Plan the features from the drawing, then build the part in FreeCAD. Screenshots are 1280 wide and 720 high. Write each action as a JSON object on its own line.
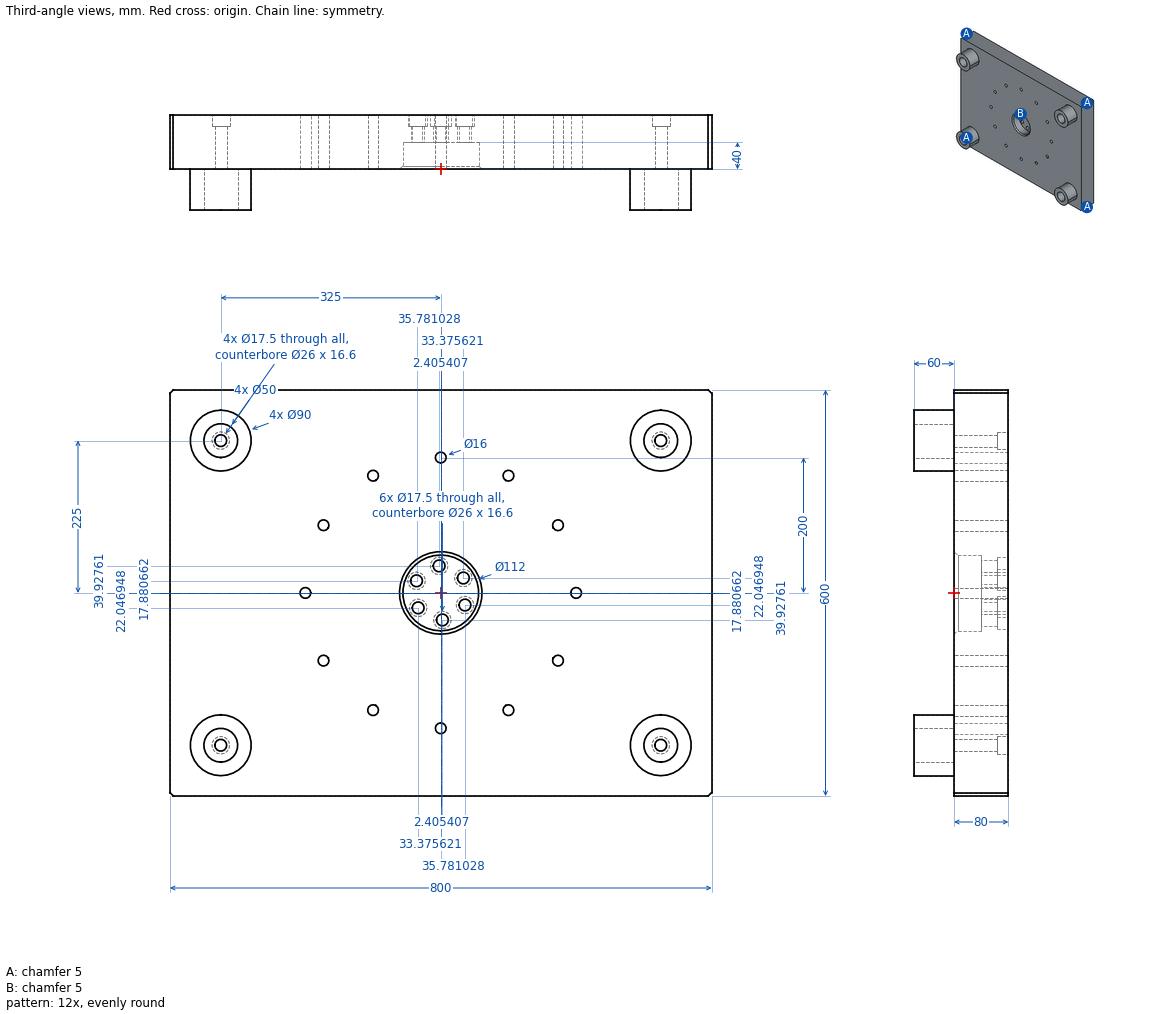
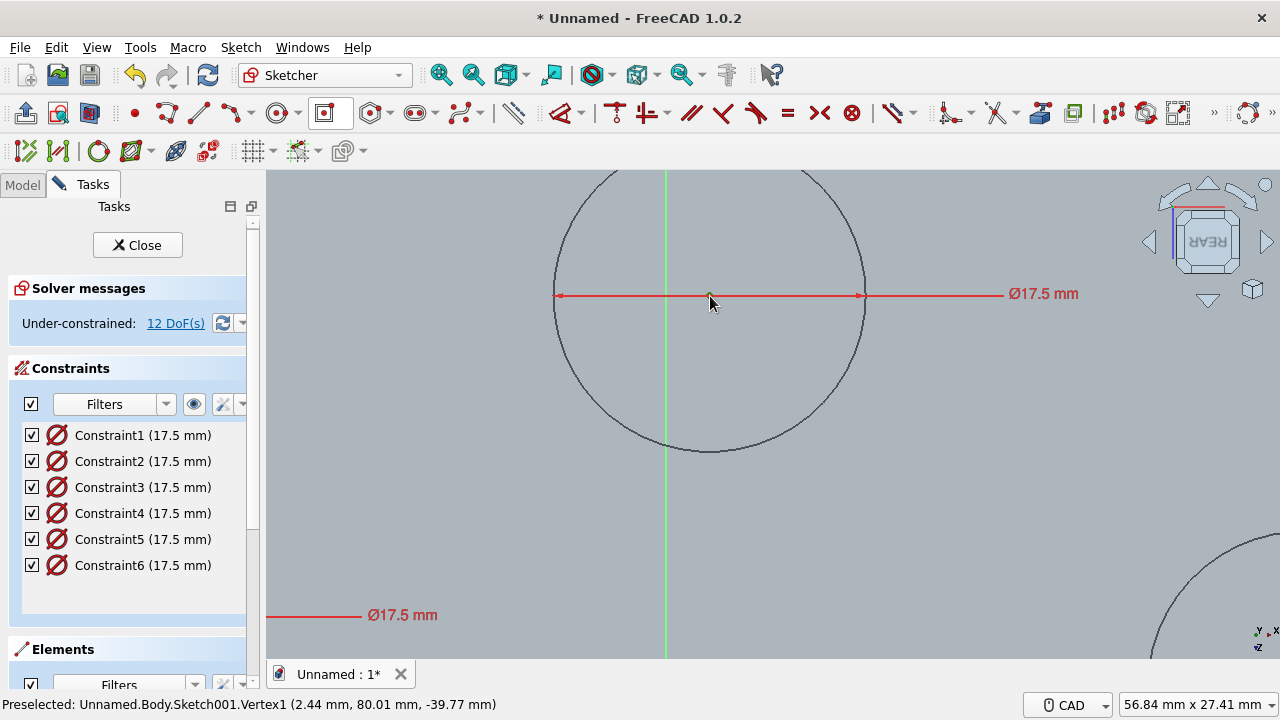
{"action": "key", "text": "l"}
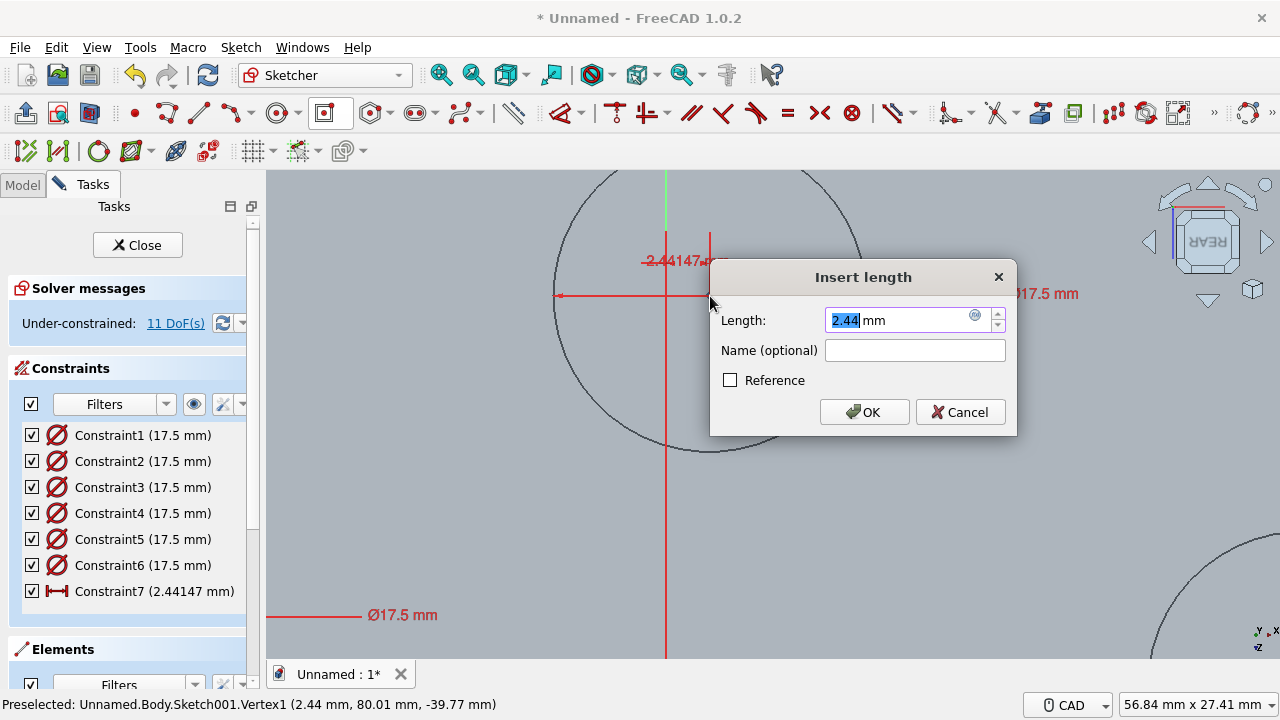
{"action": "type", "text": "2.405407"}
{"action": "key", "text": "Return"}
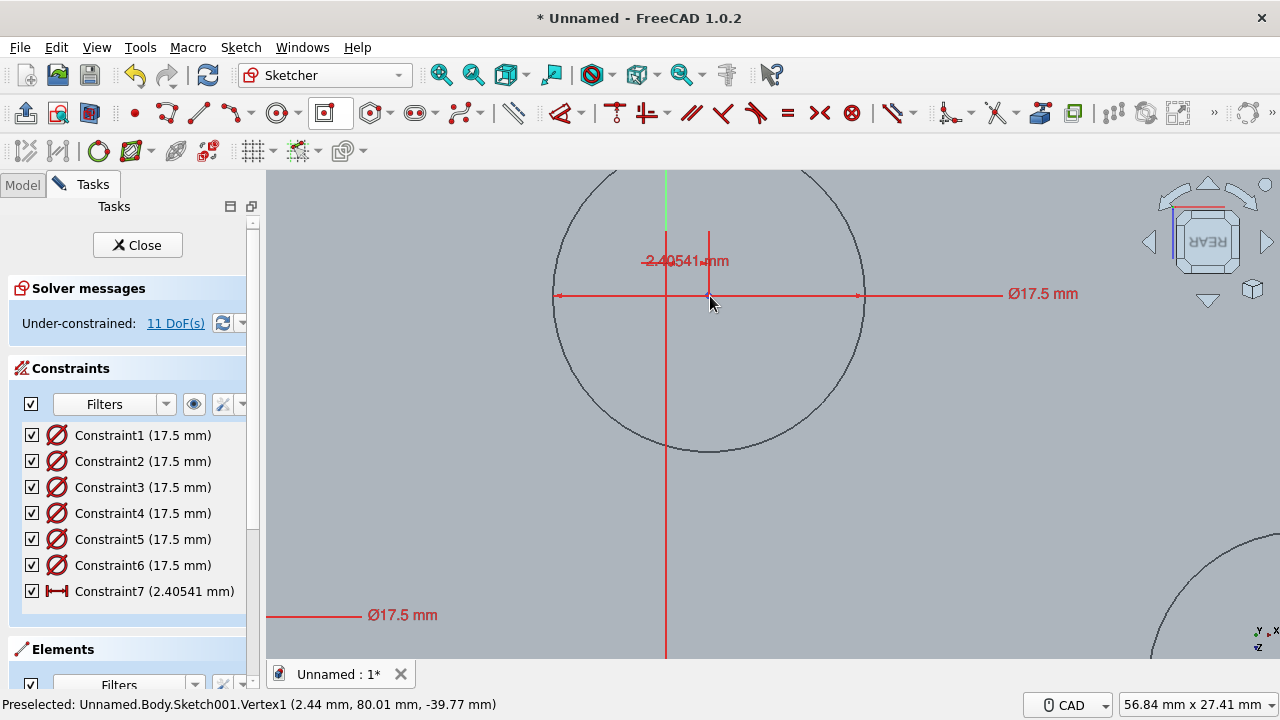
{"action": "scroll", "coordinate": [712, 297], "scroll_direction": "down", "scroll_amount": 9}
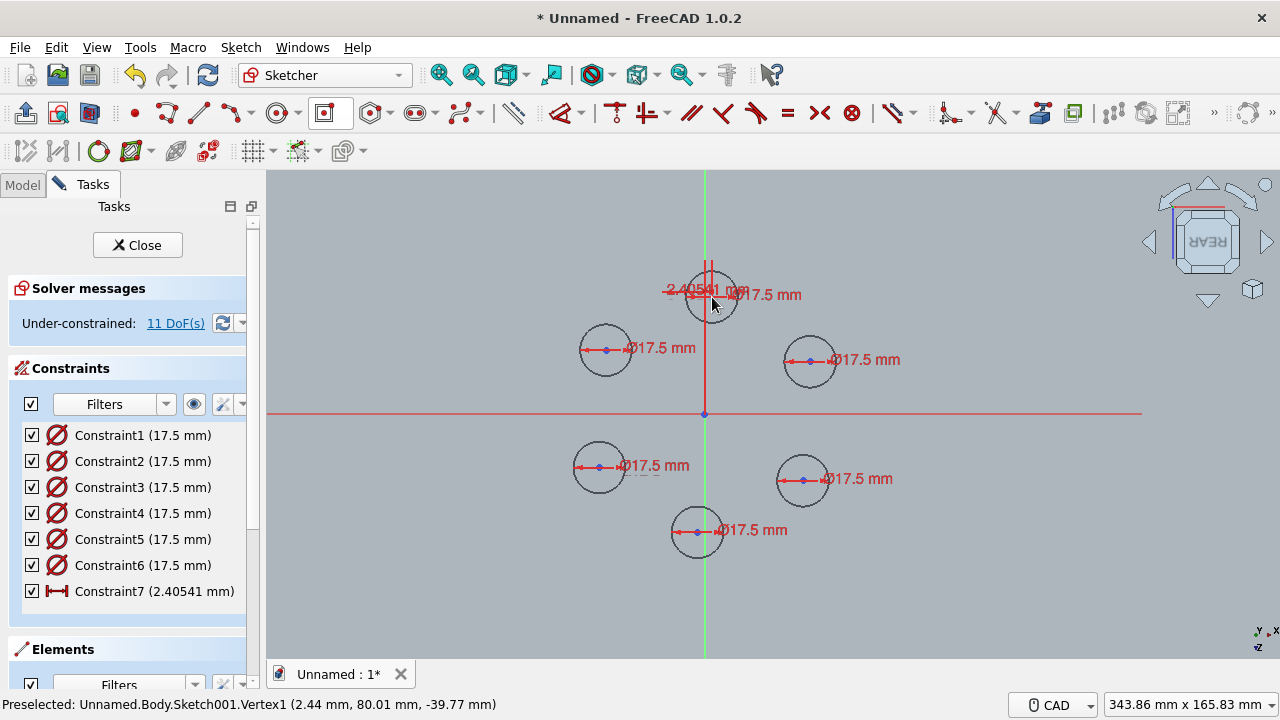
{"action": "left_click", "coordinate": [712, 297]}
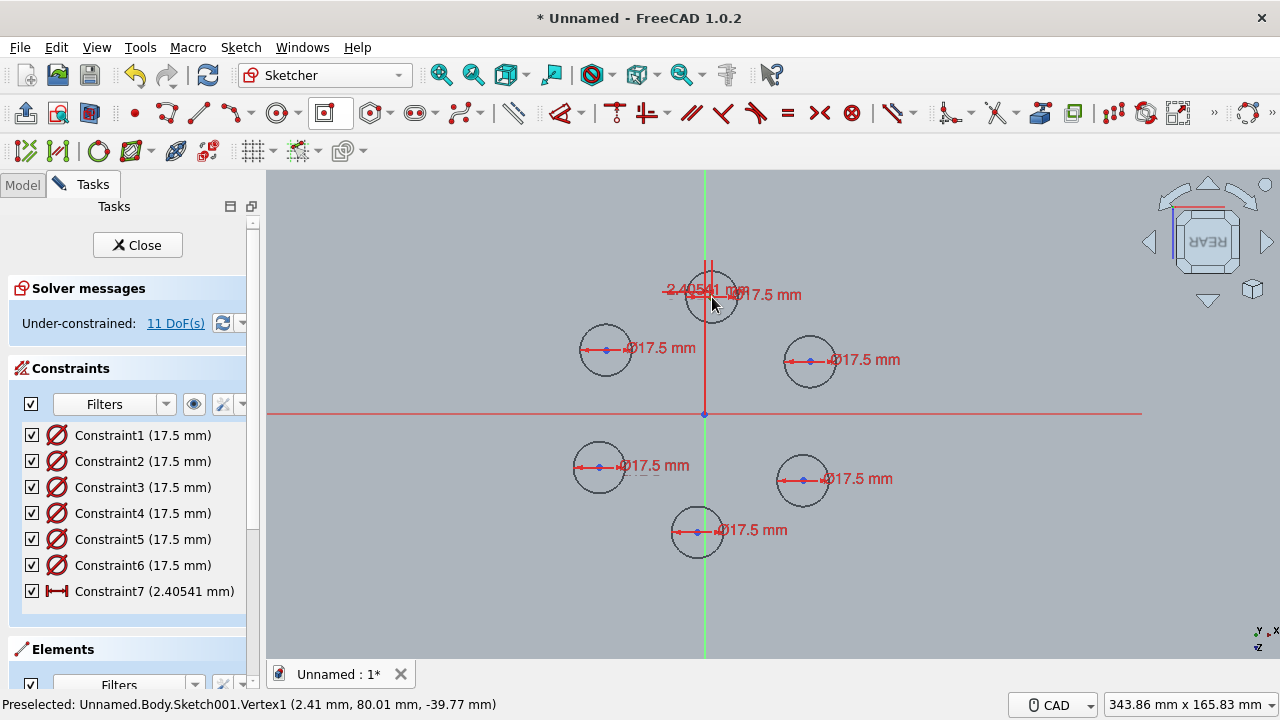
{"action": "key", "text": "i"}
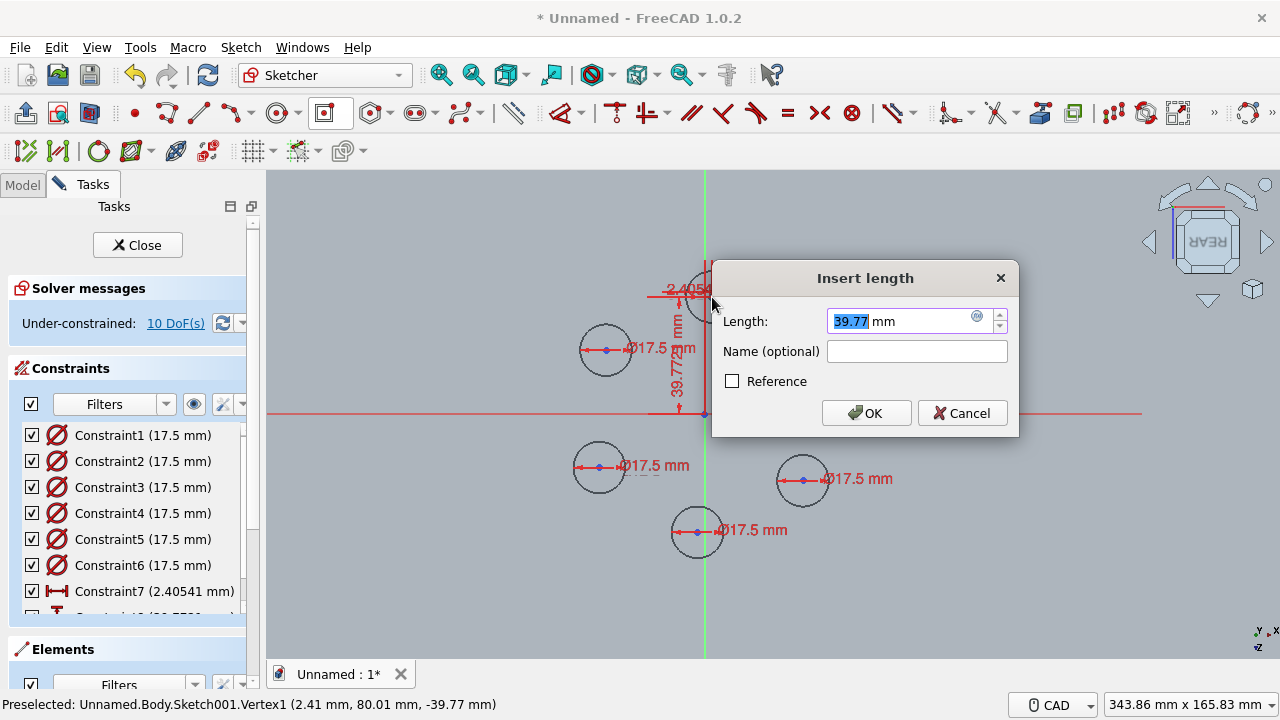
{"action": "type", "text": "39.92761"}
{"action": "key", "text": "Return"}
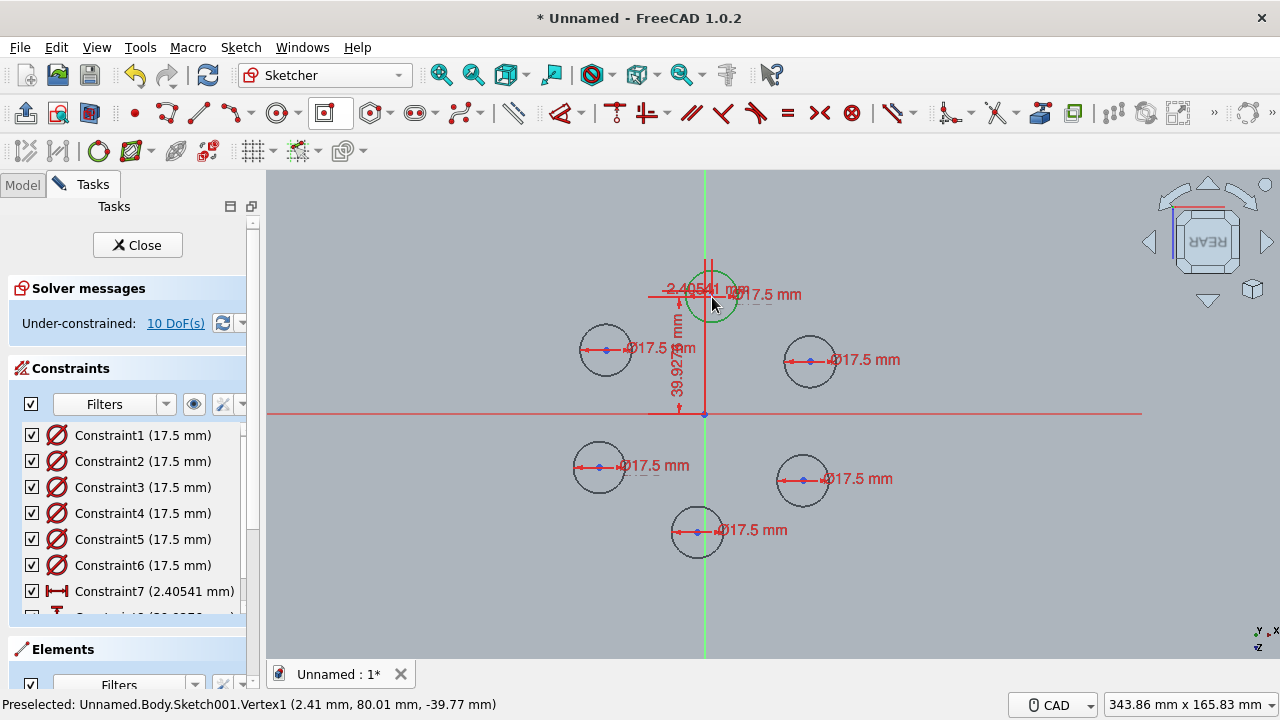
{"action": "scroll", "coordinate": [698, 532], "scroll_direction": "up", "scroll_amount": 9}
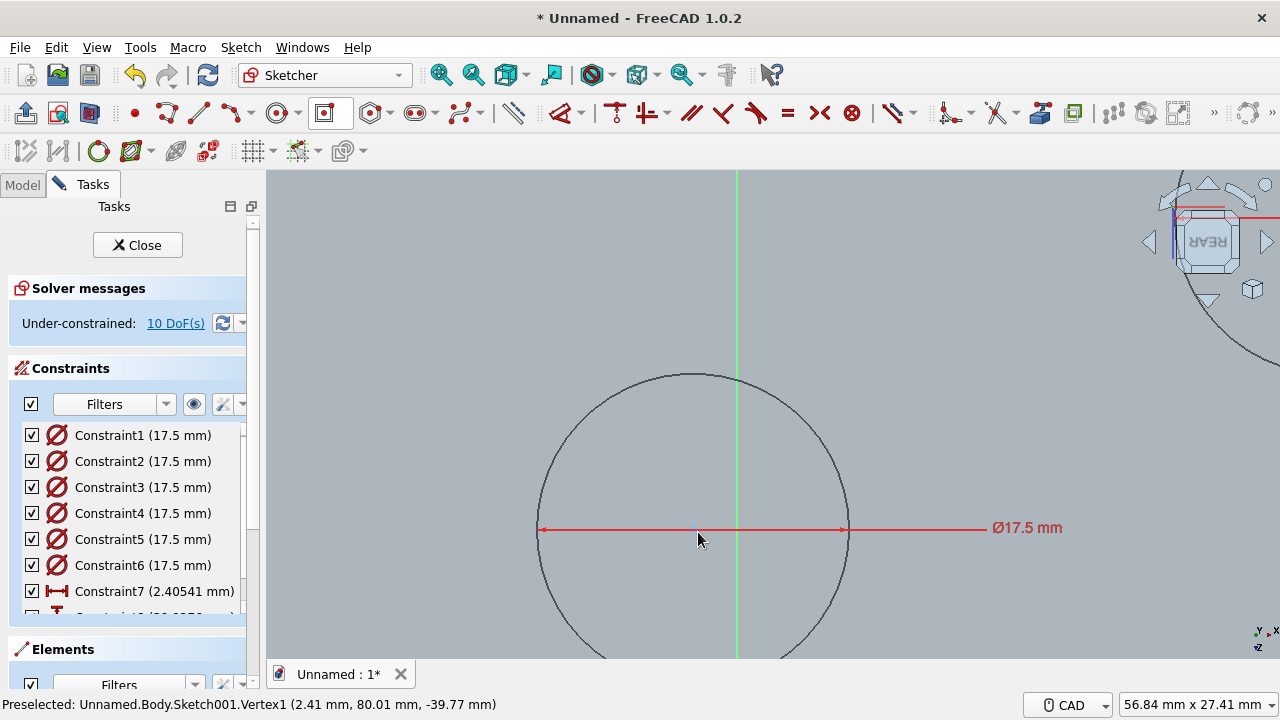
{"action": "left_click", "coordinate": [693, 530]}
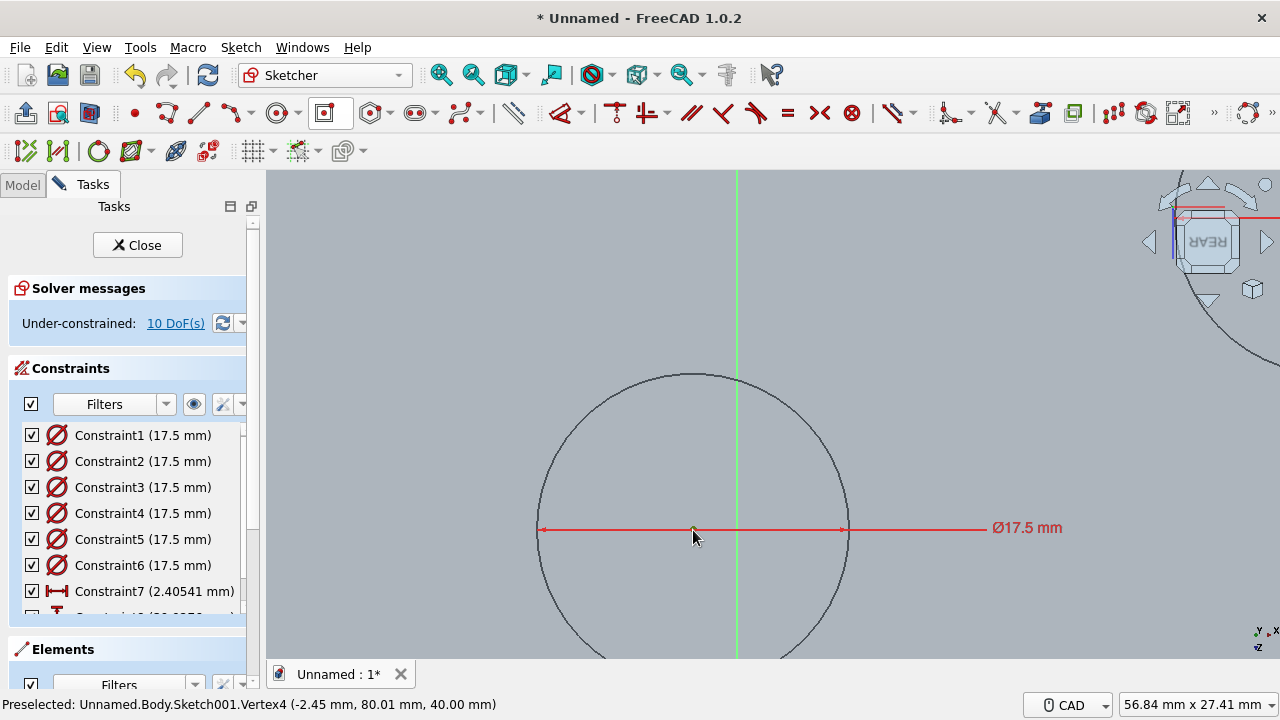
{"action": "key", "text": "l"}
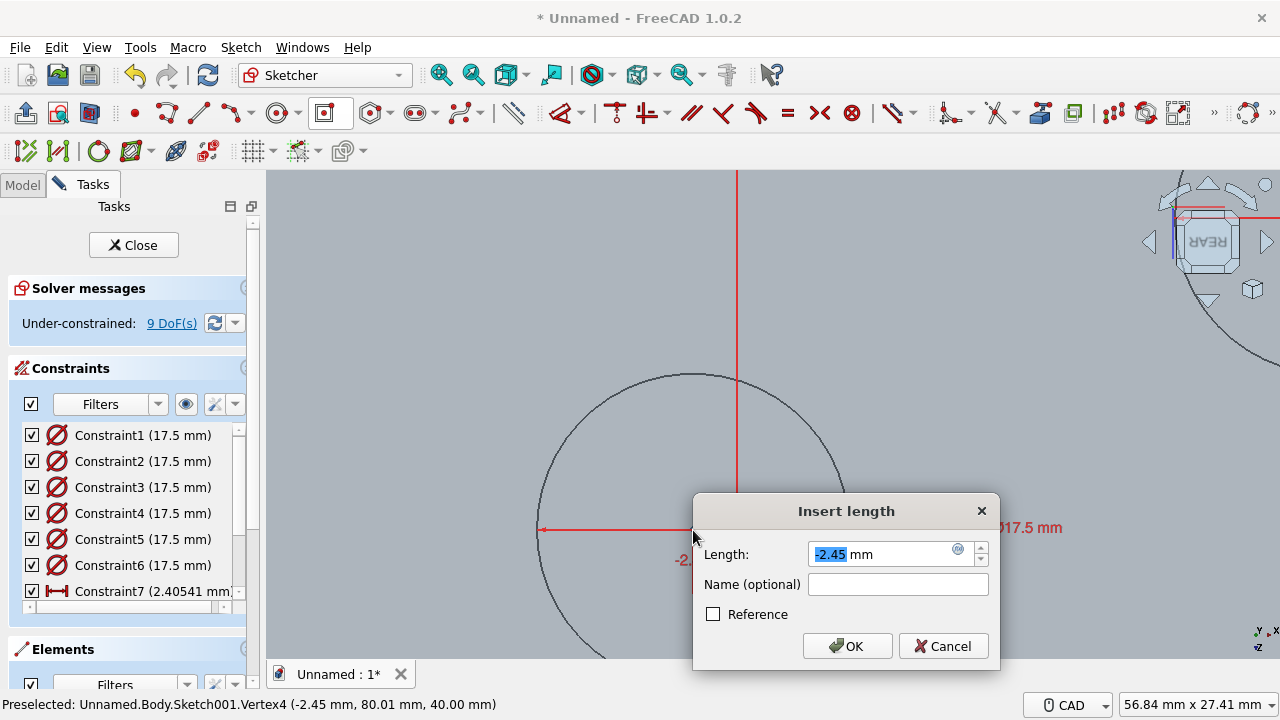
{"action": "type", "text": "-2.405407"}
{"action": "key", "text": "Return"}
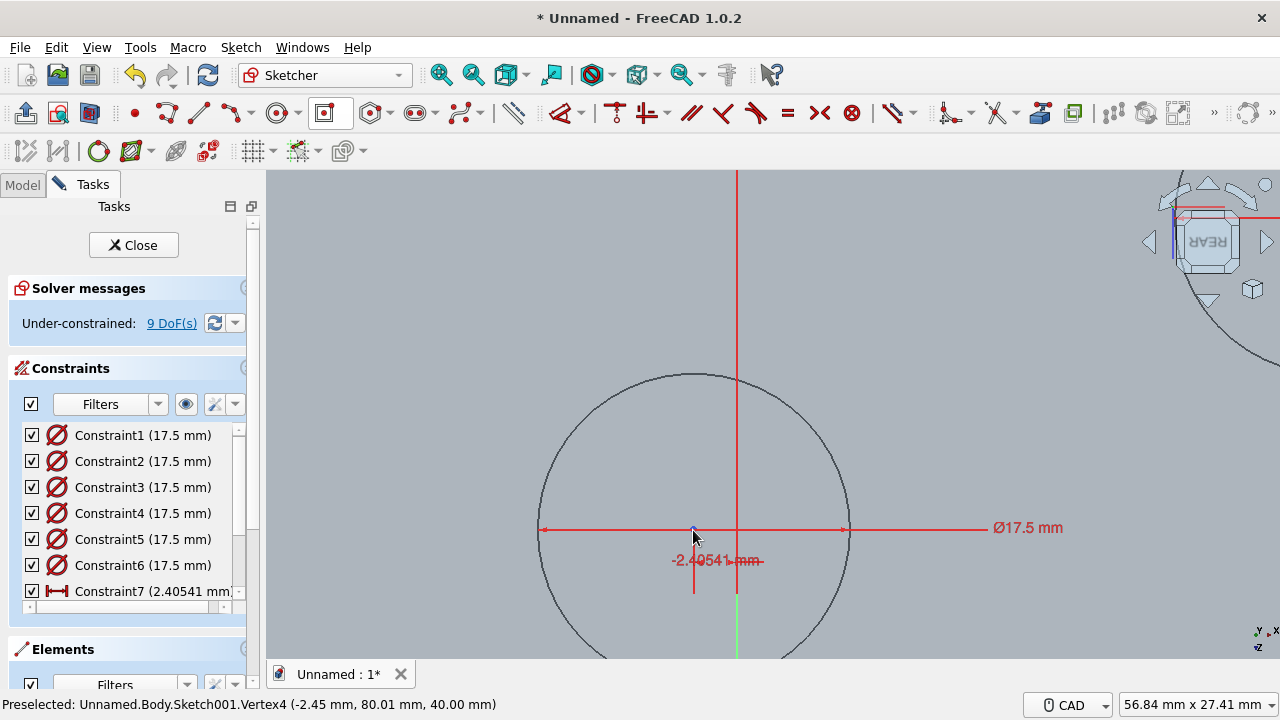
{"action": "scroll", "coordinate": [698, 533], "scroll_direction": "down", "scroll_amount": 9}